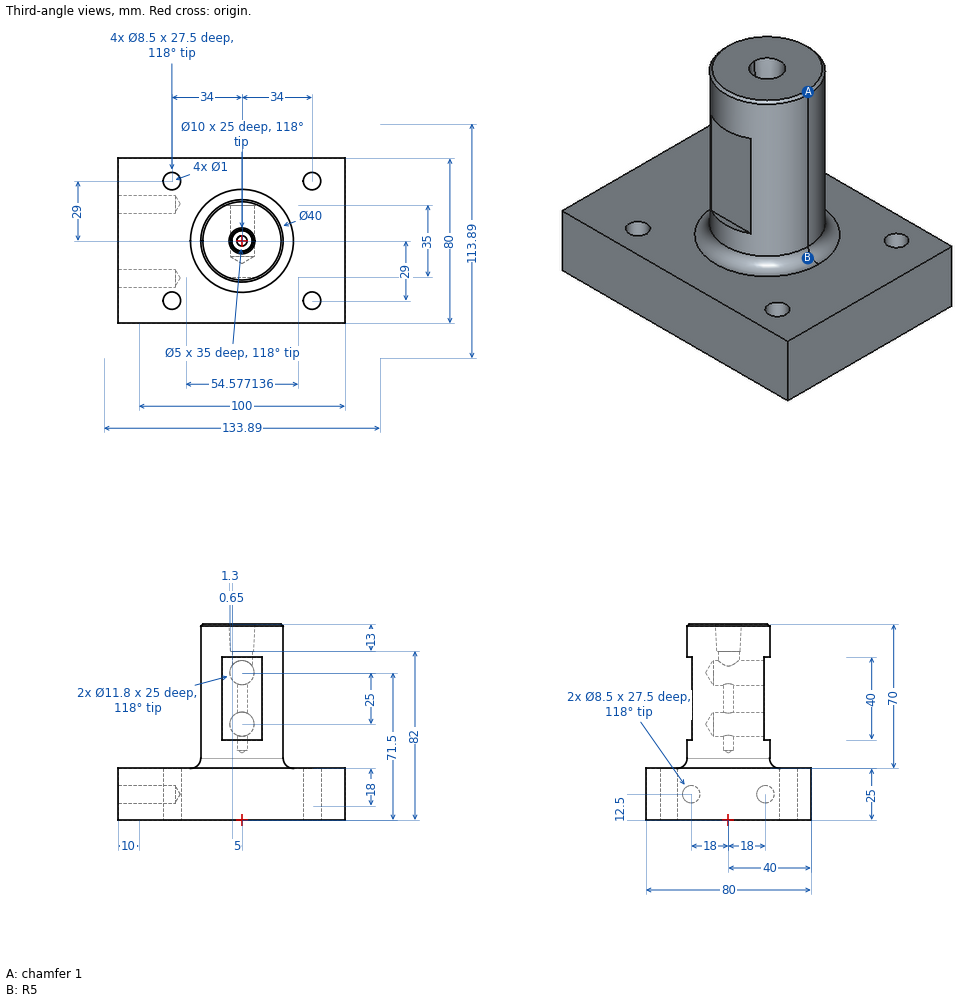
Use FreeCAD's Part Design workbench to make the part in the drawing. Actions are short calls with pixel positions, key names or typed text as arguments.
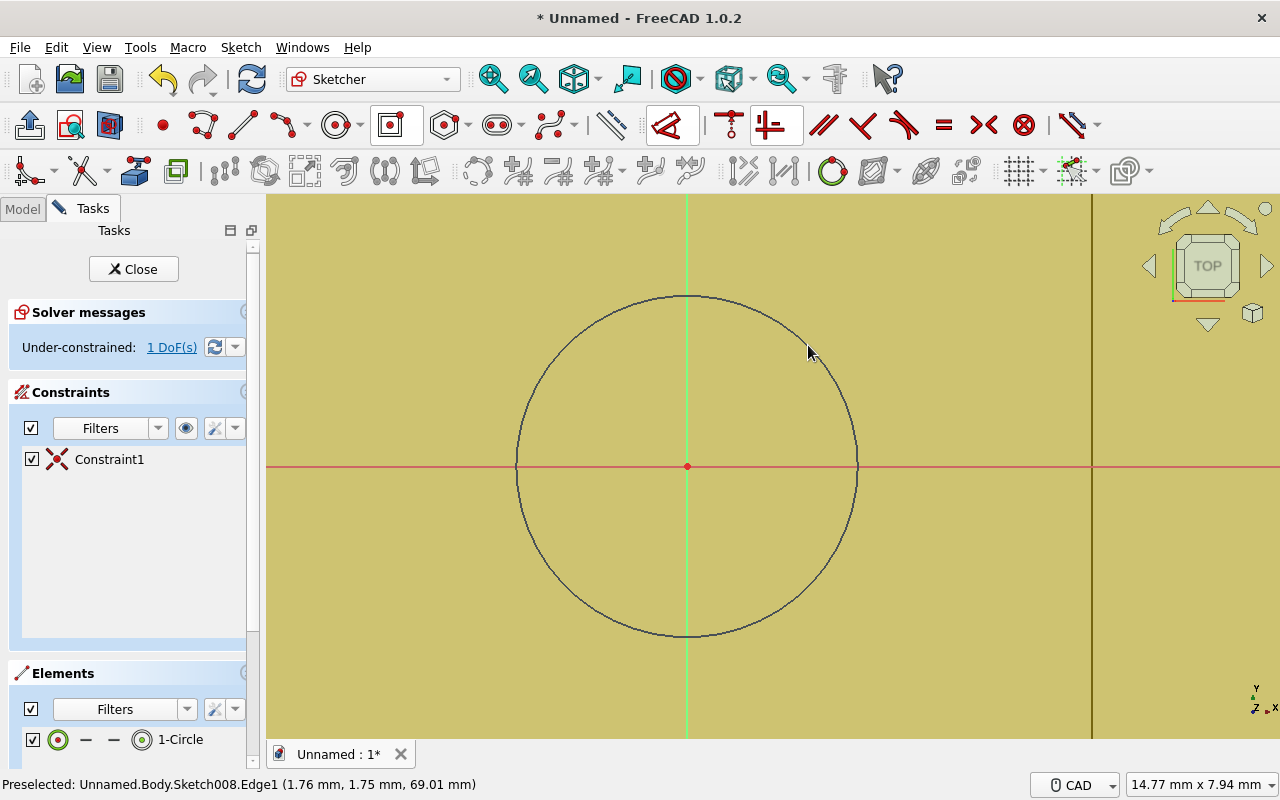
click(807, 345)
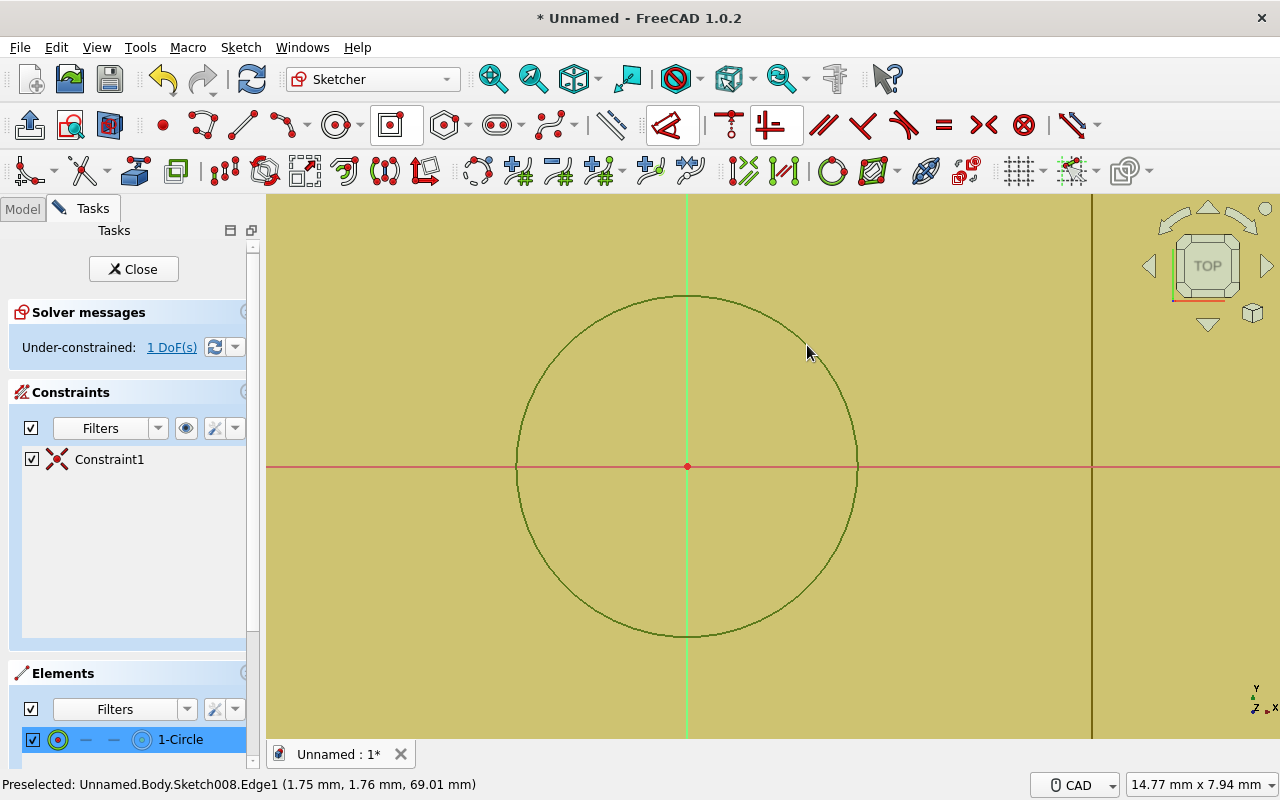
key(k)
key(o)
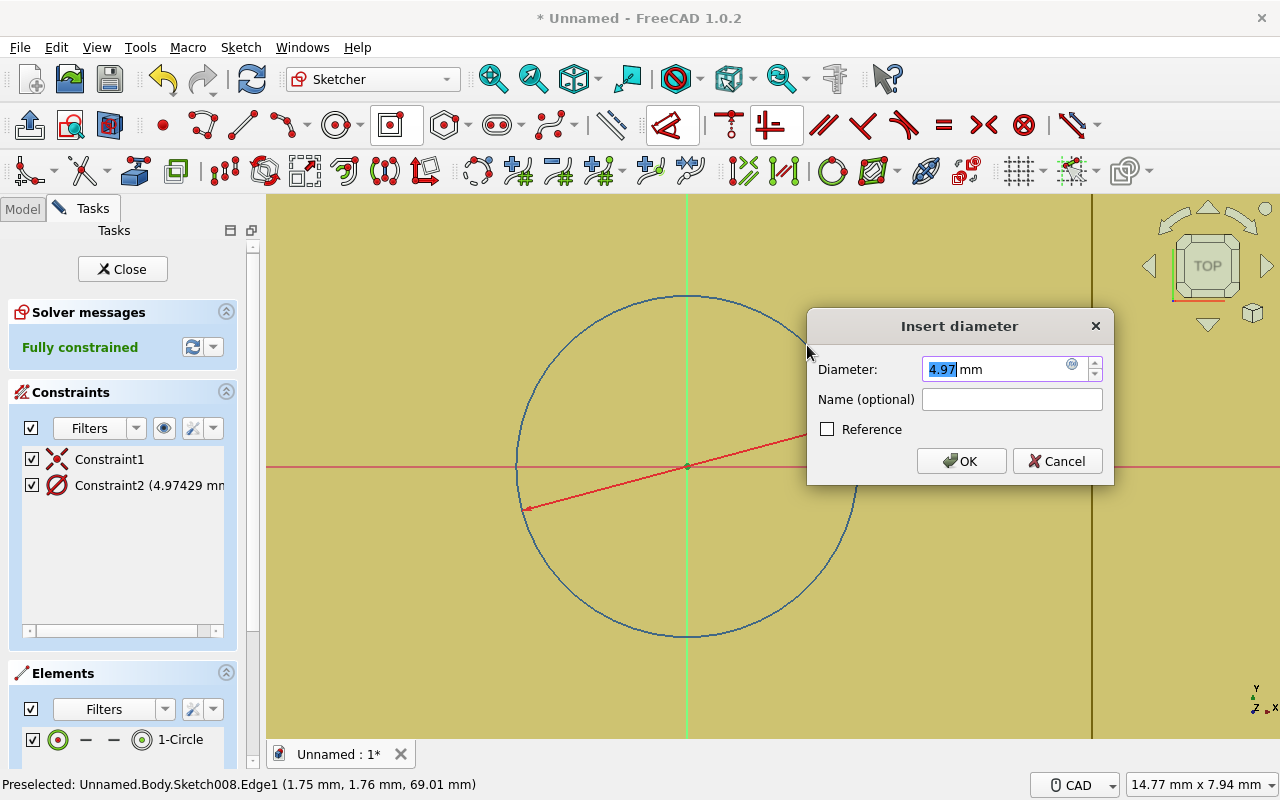
text(5)
key(Return)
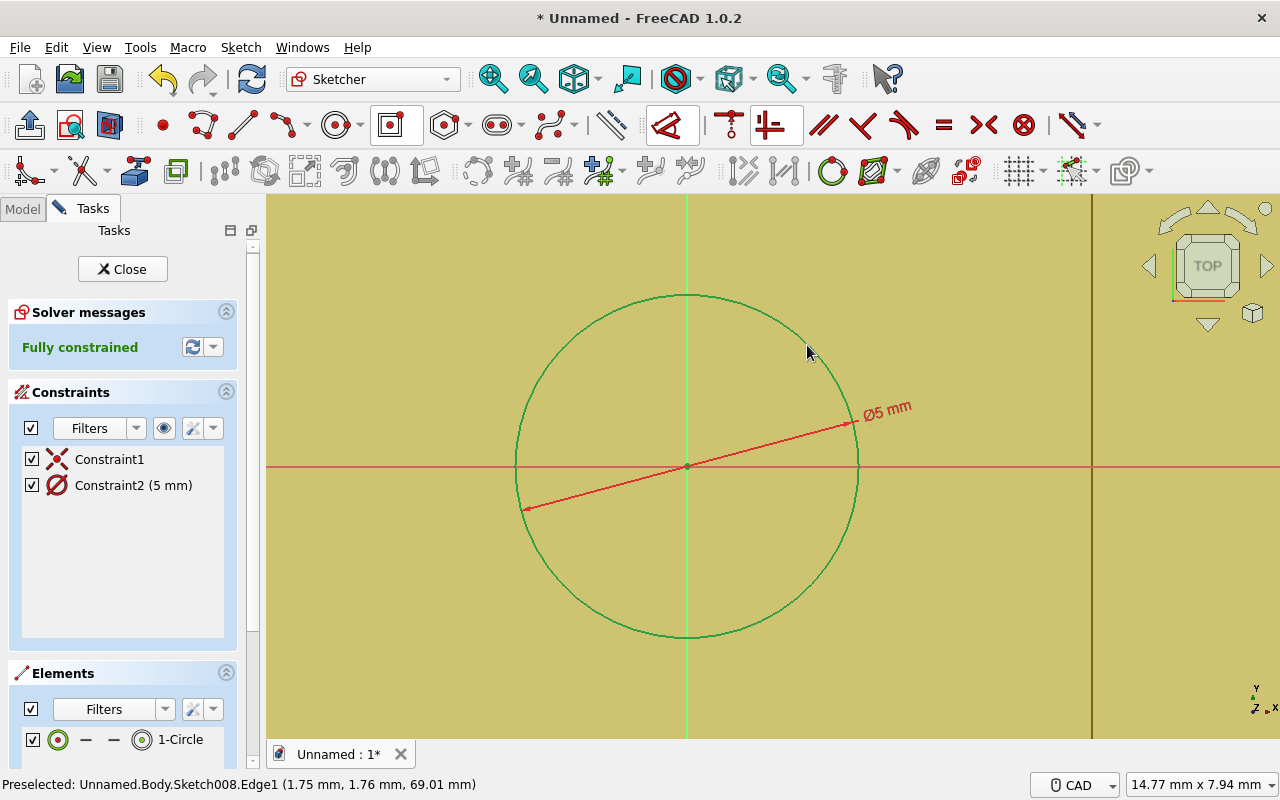
click(123, 269)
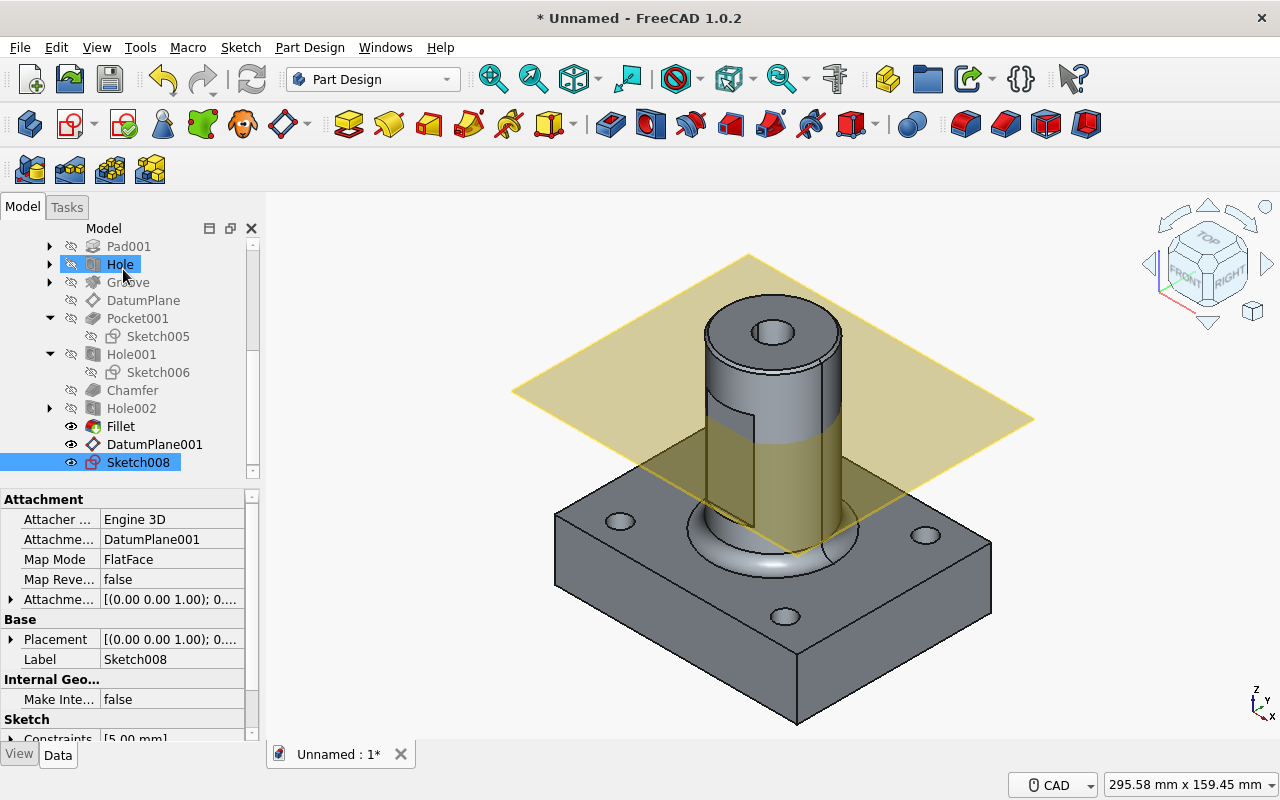
click(652, 124)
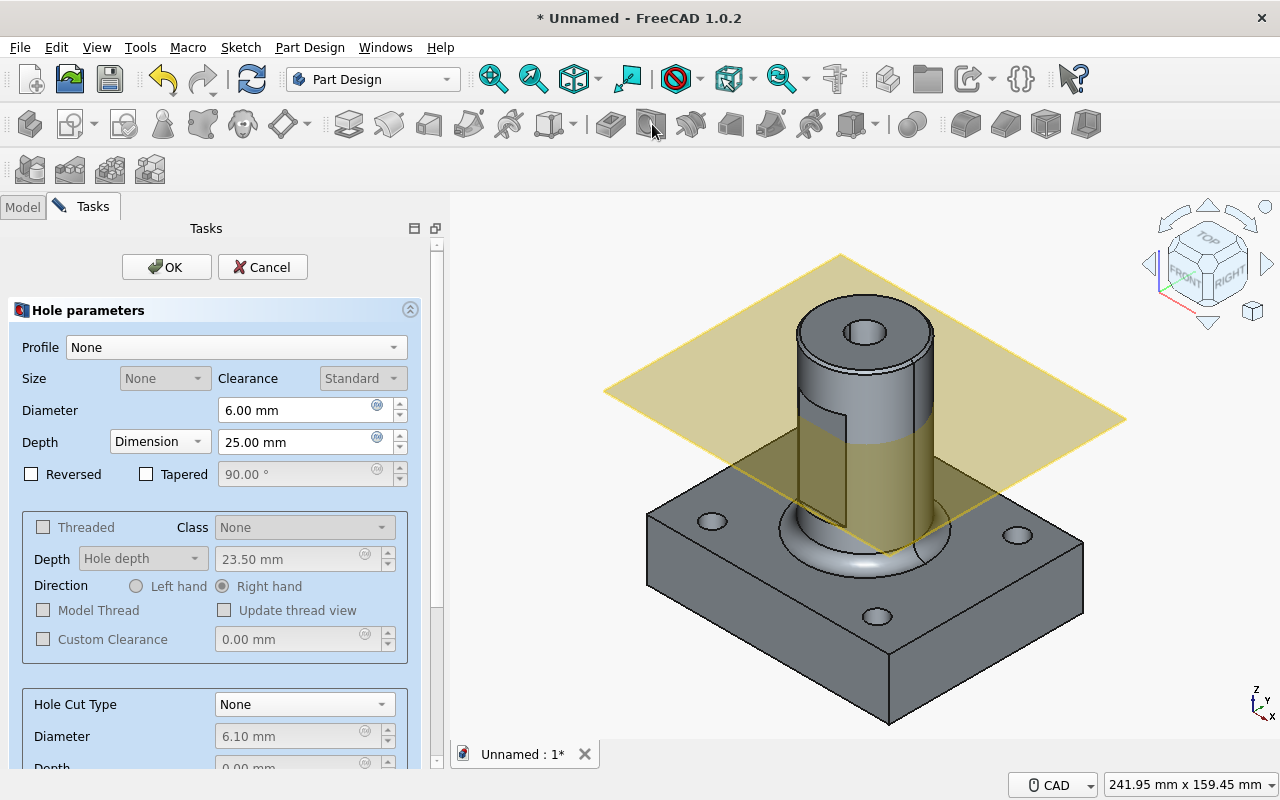
triple_click(305, 410)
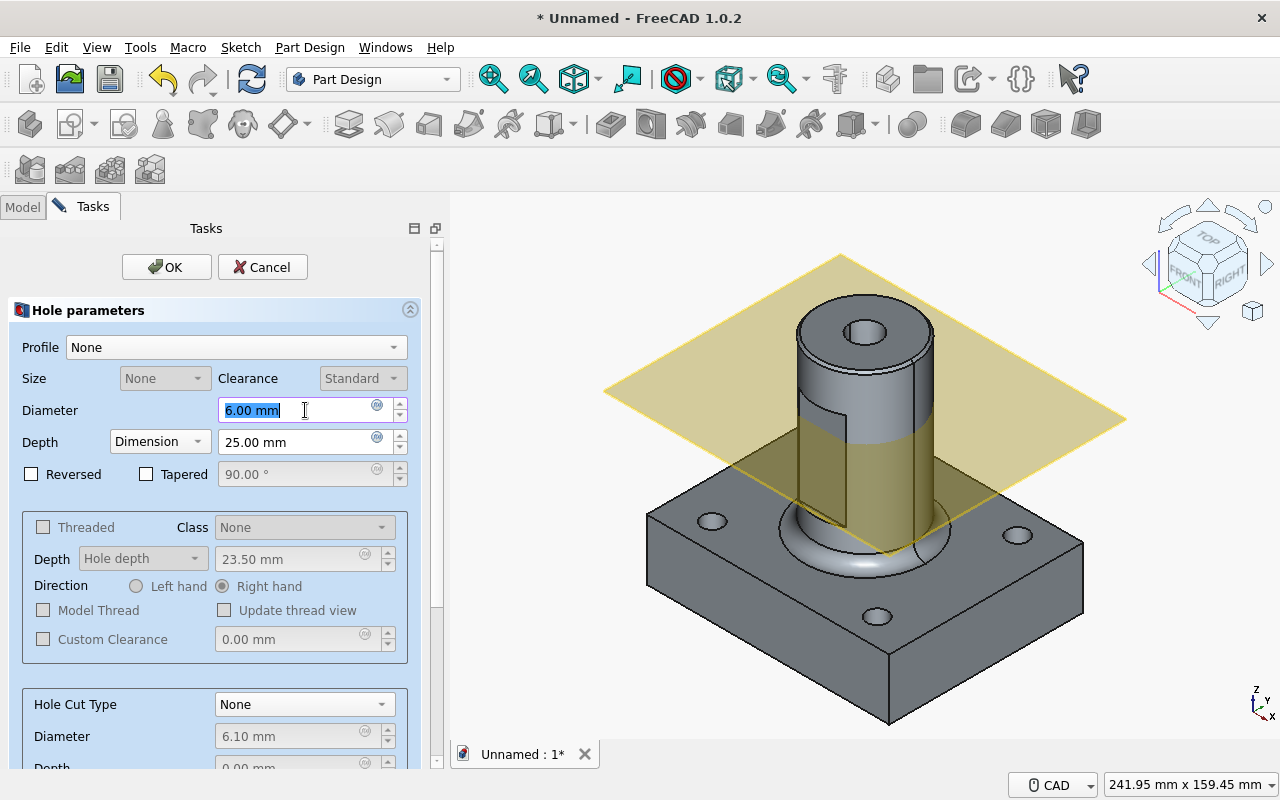
text(5)
key(Tab)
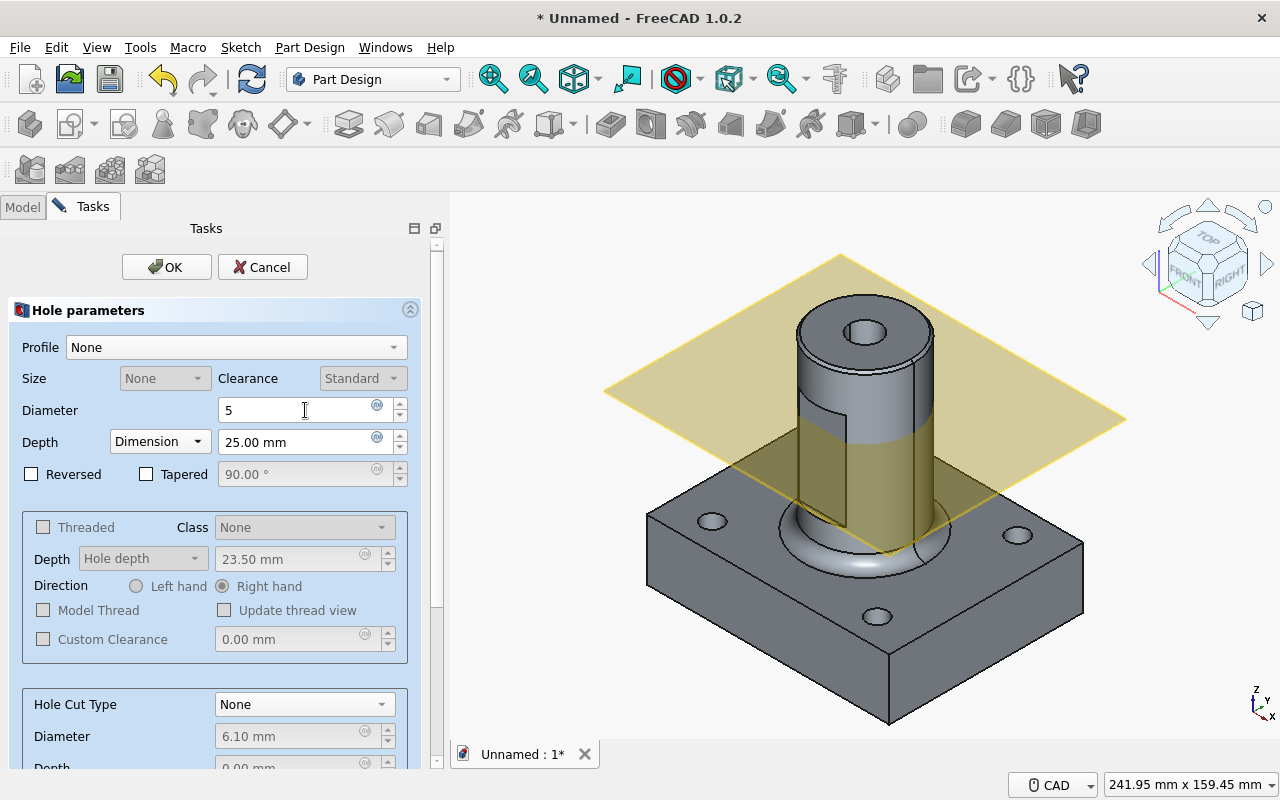
triple_click(305, 442)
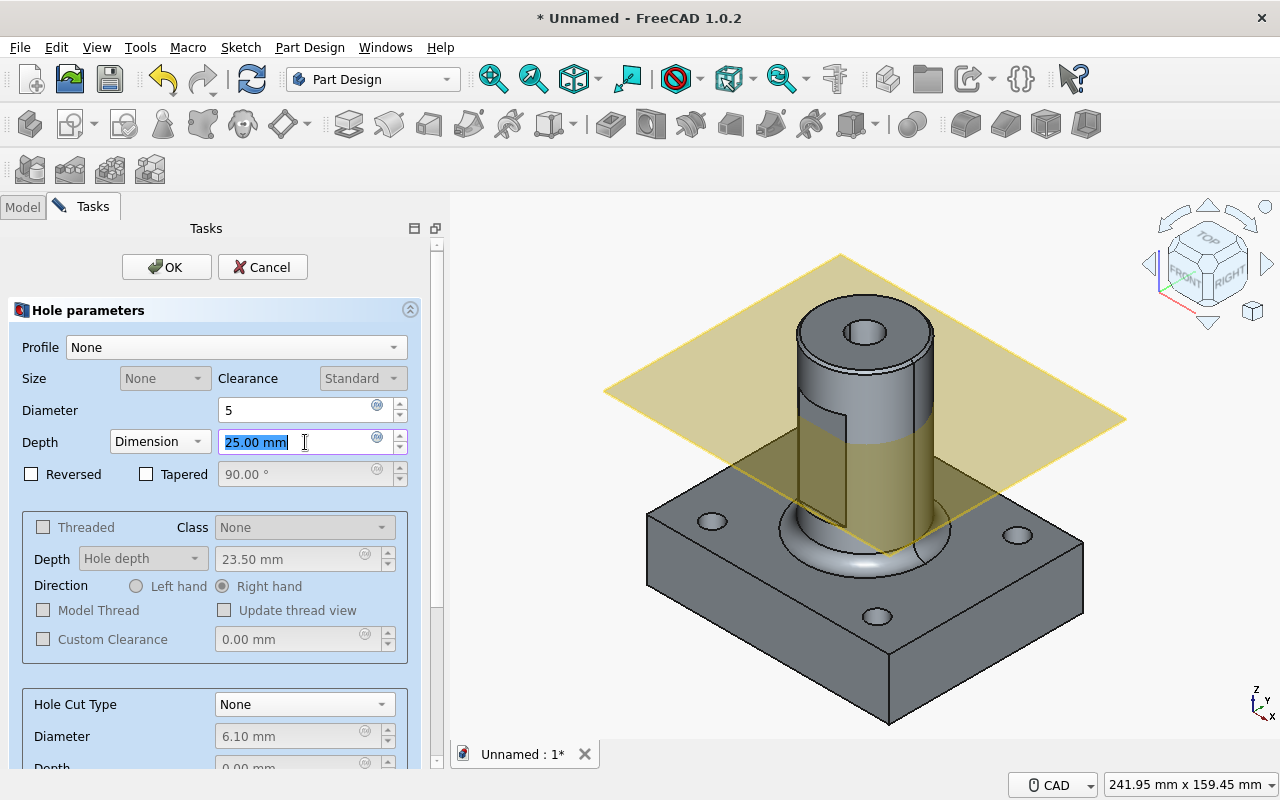
text(35)
key(Tab)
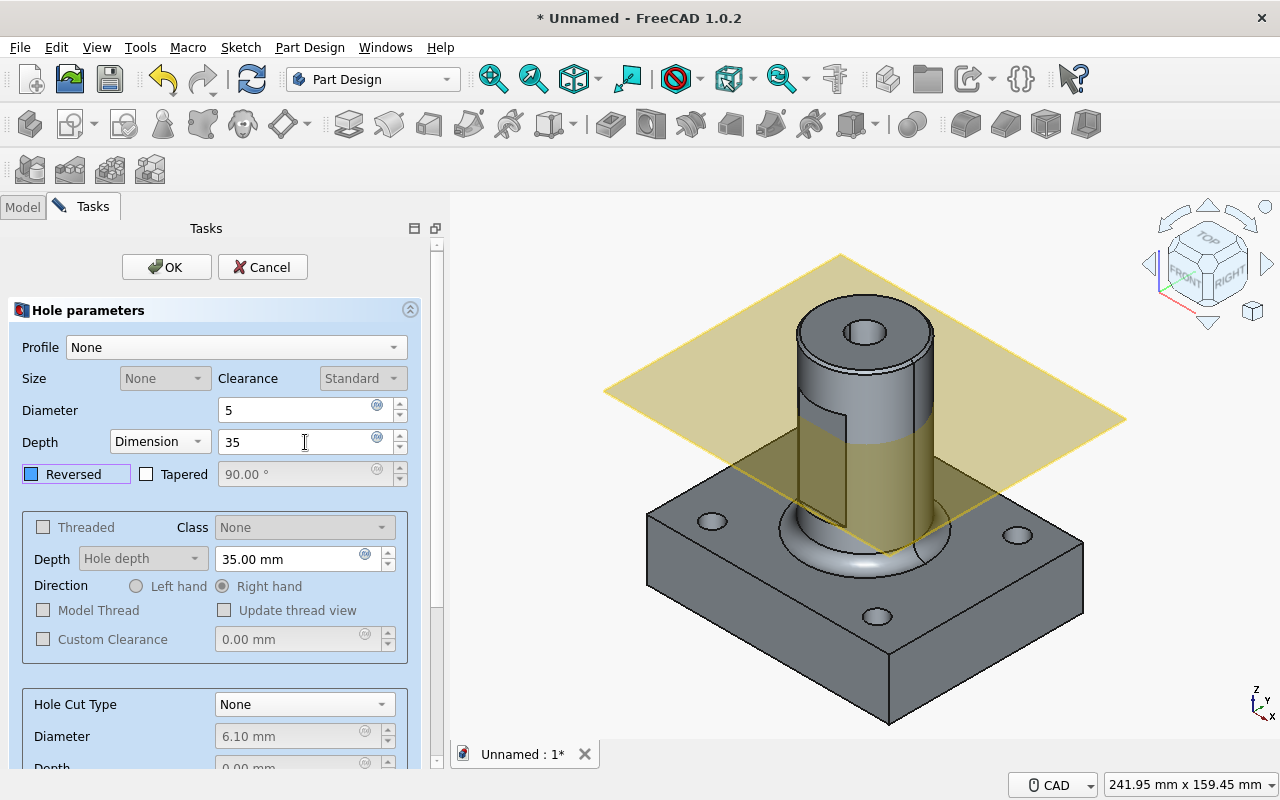
click(167, 267)